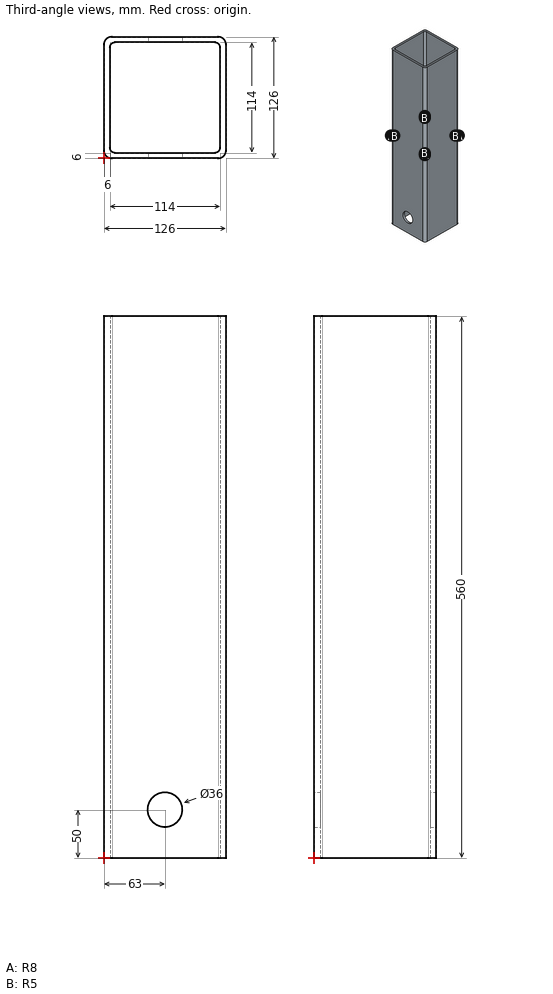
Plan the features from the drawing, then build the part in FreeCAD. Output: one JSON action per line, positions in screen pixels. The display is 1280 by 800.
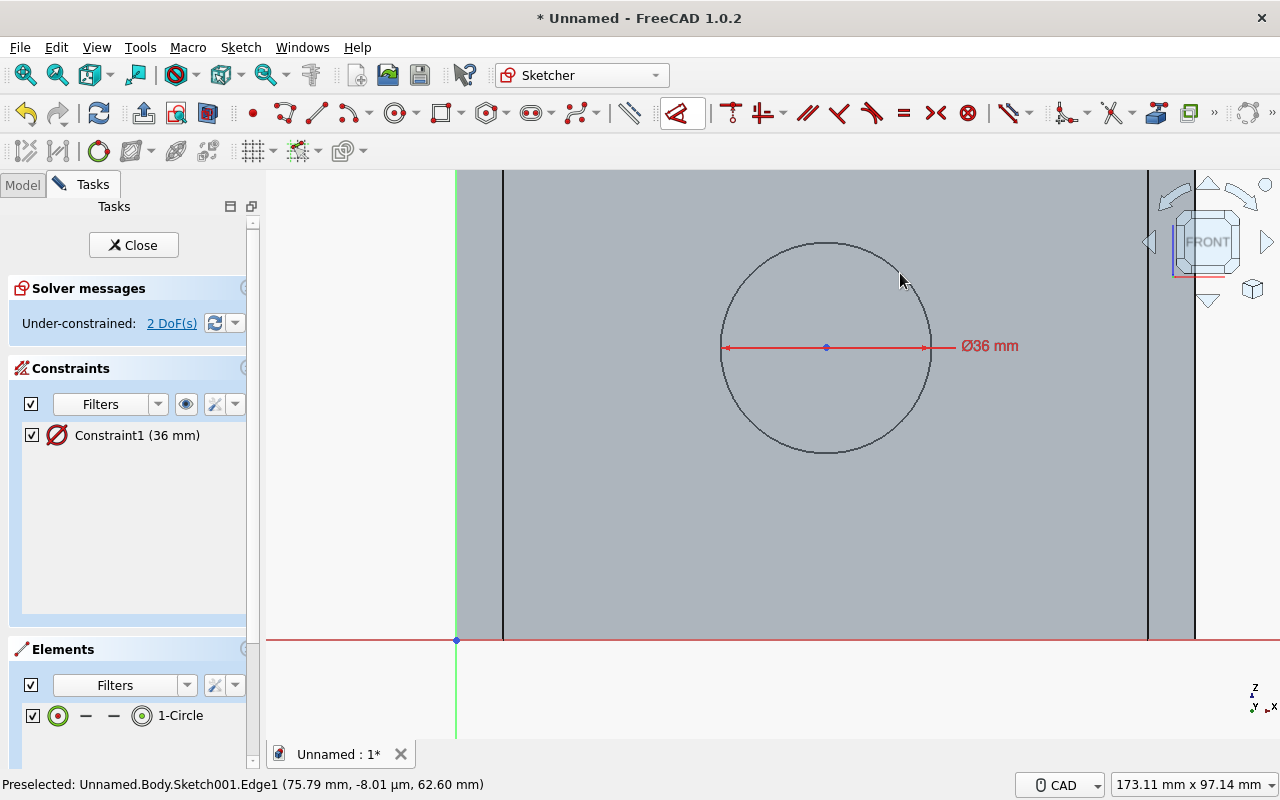
{"action": "left_click", "coordinate": [826, 348]}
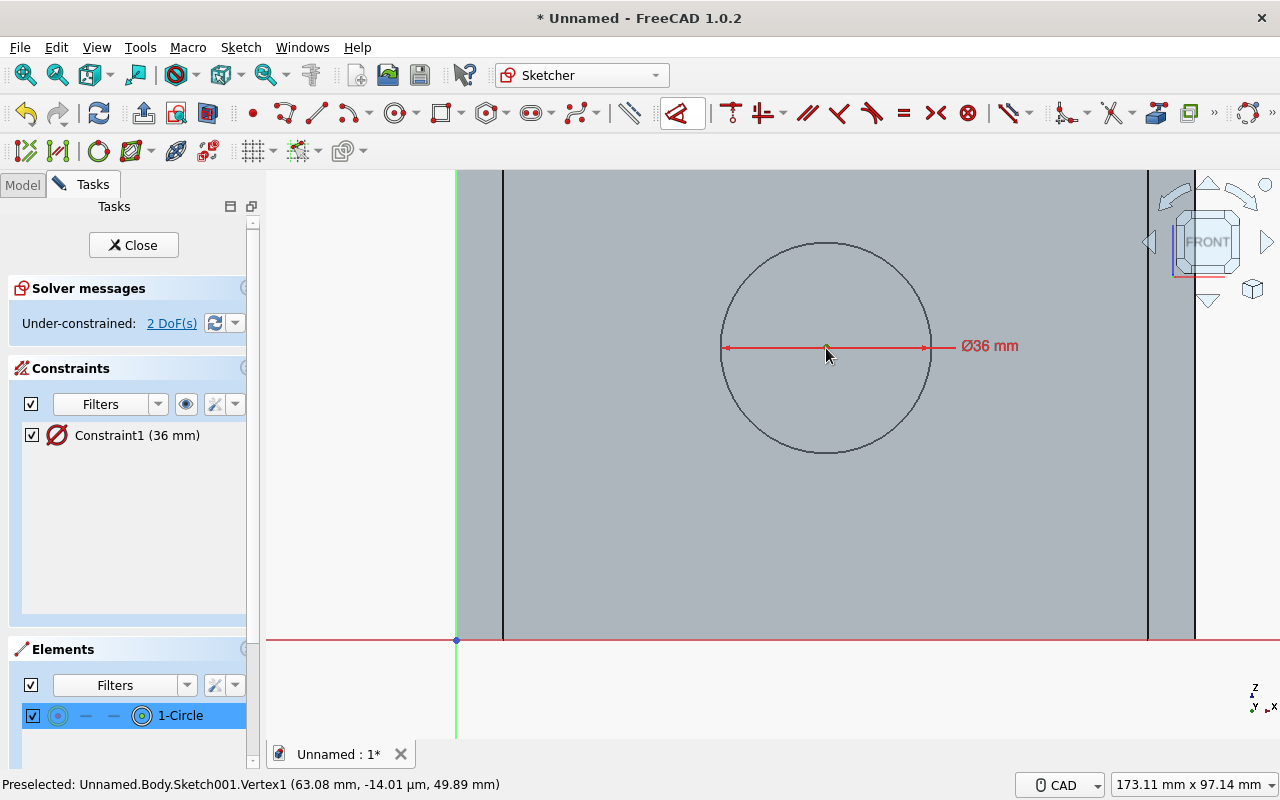
{"action": "left_click", "coordinate": [700, 114]}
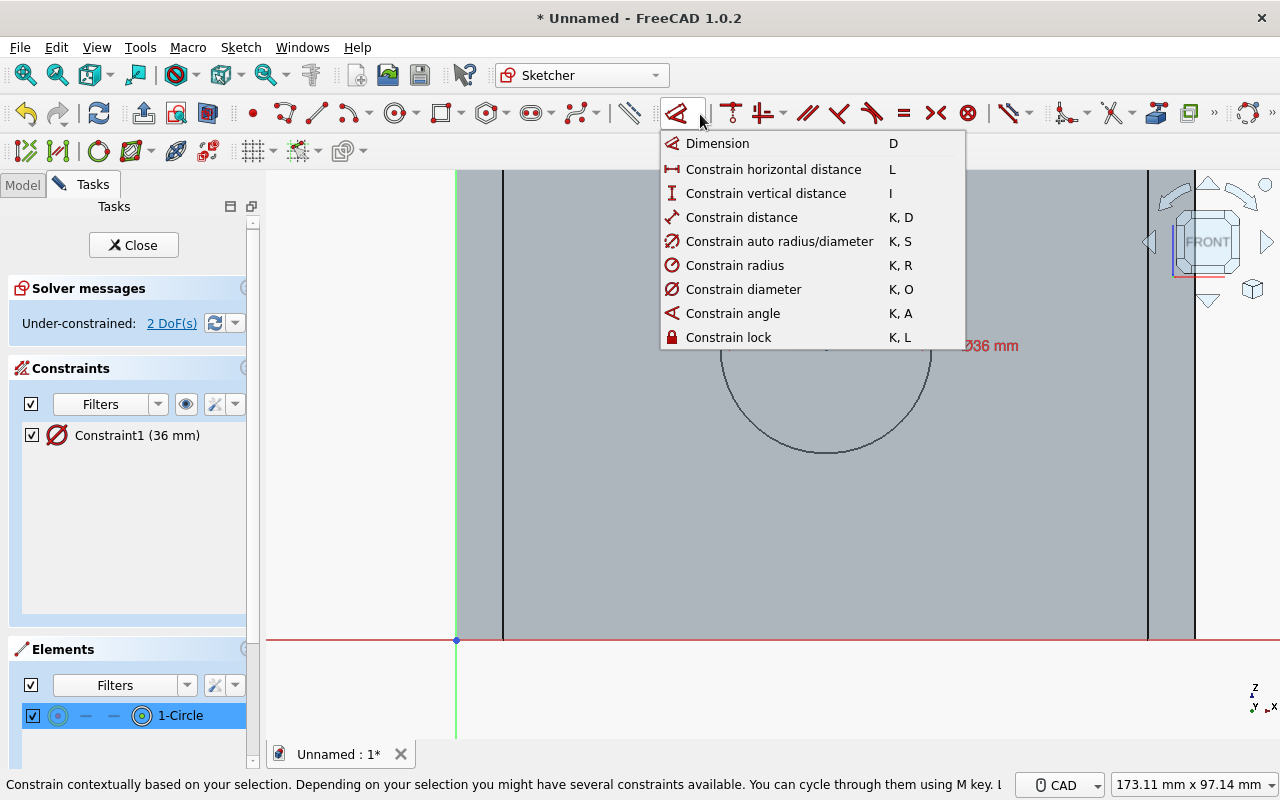
{"action": "left_click", "coordinate": [813, 169]}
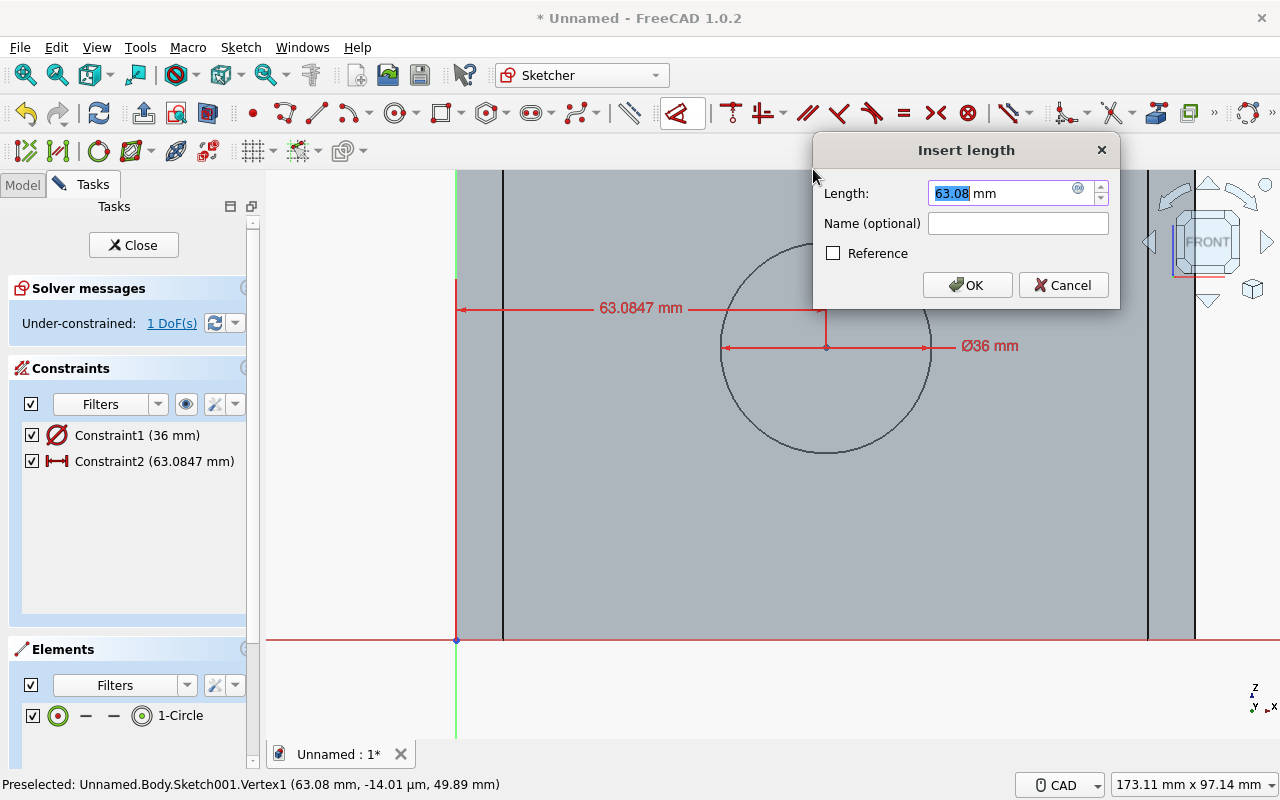
{"action": "type", "text": "63"}
{"action": "key", "text": "Return"}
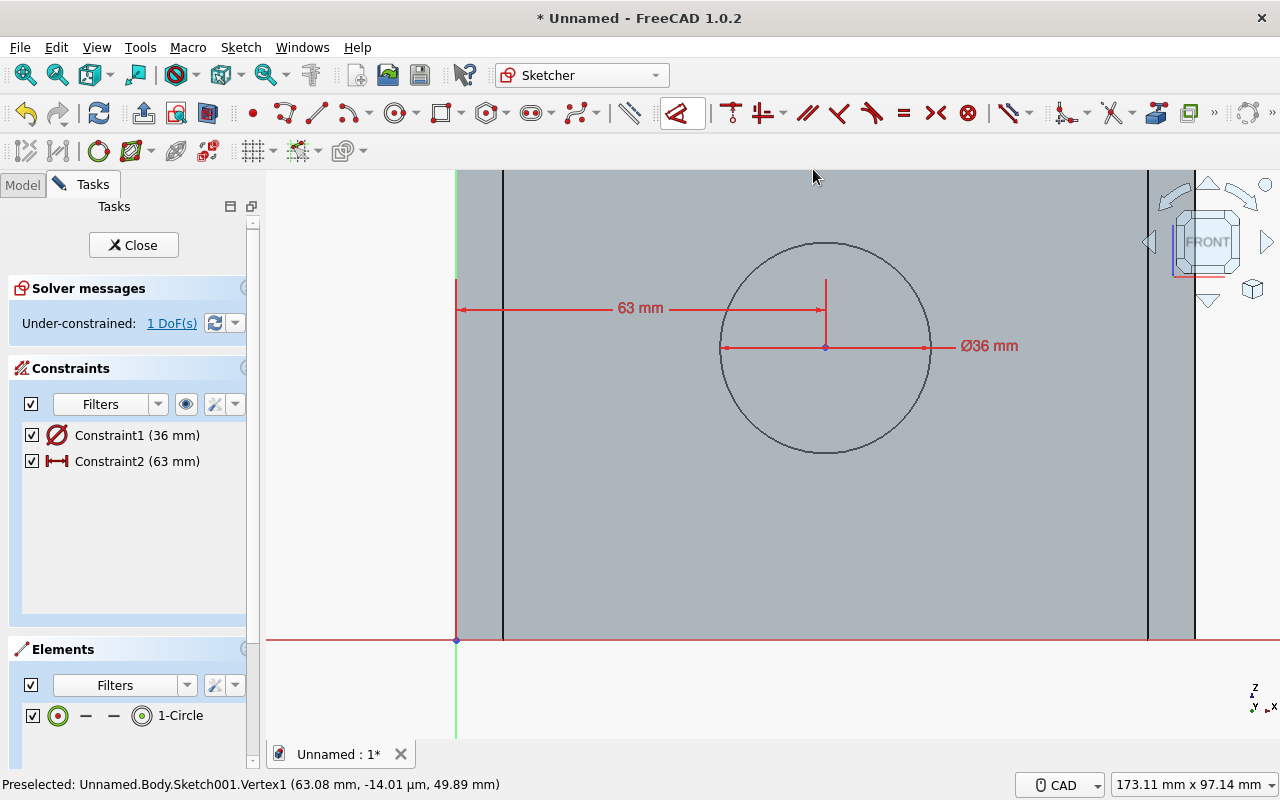
{"action": "left_click", "coordinate": [826, 348]}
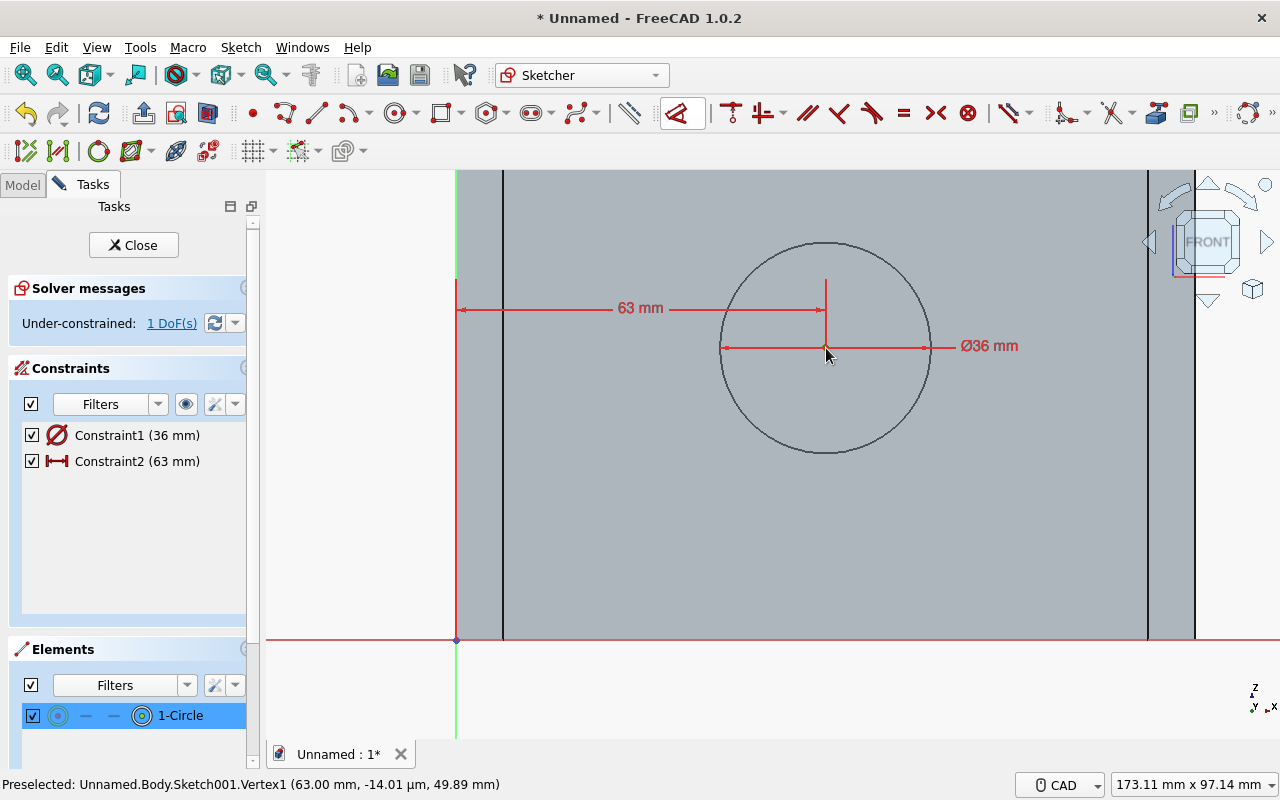
{"action": "key", "text": "i"}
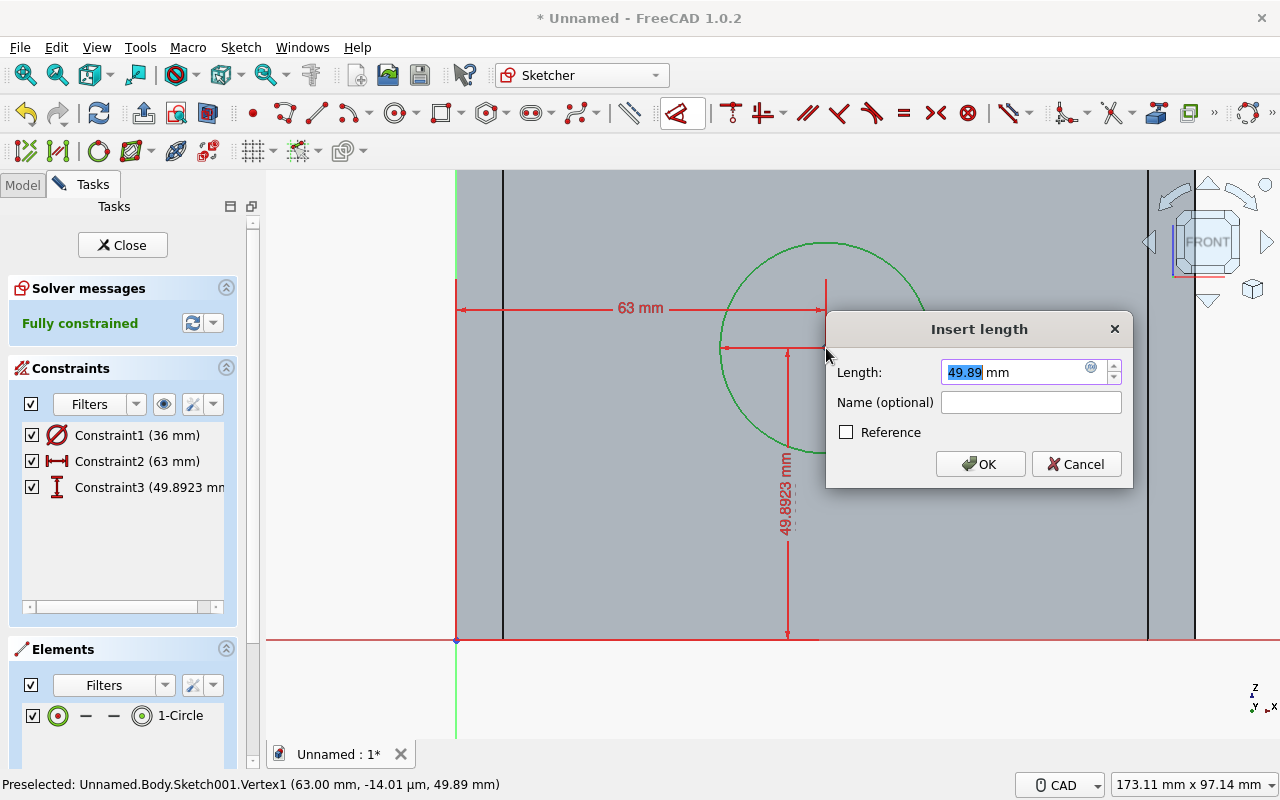
{"action": "type", "text": "50"}
{"action": "key", "text": "Return"}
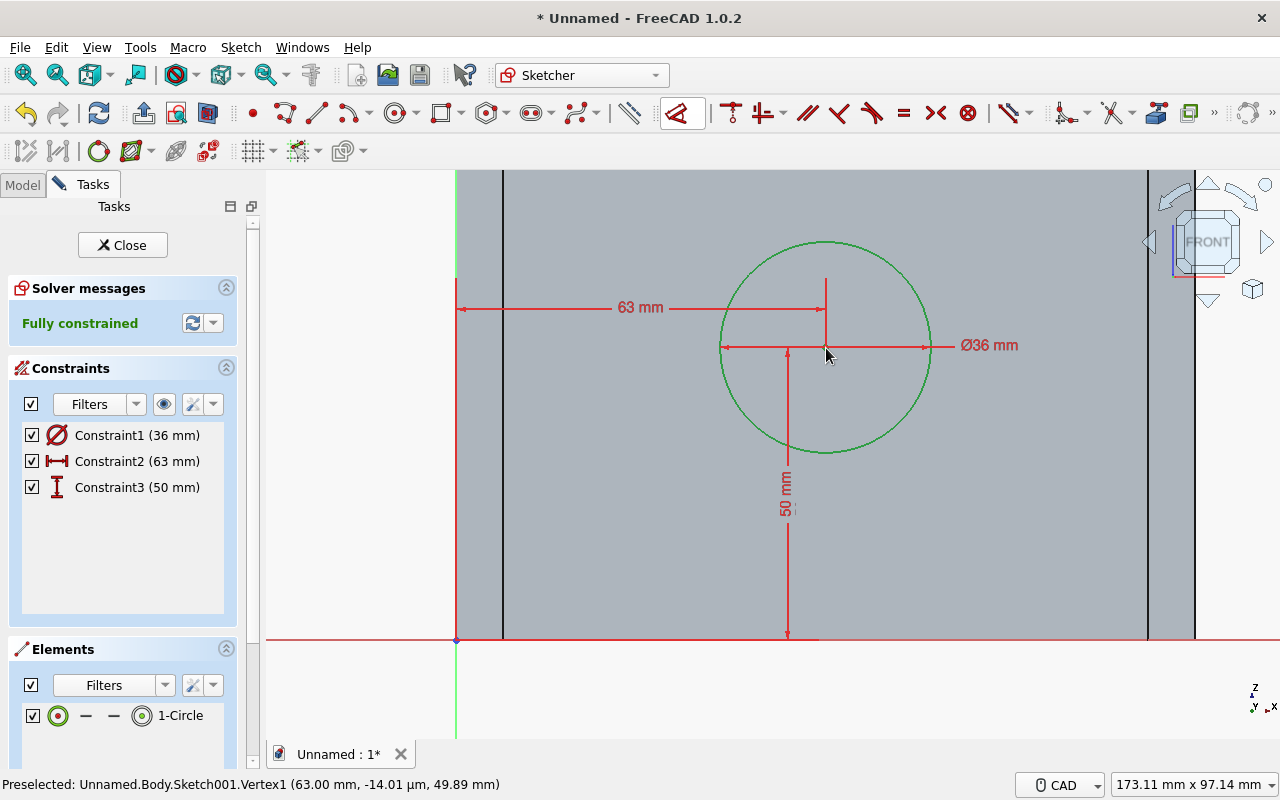
{"action": "left_click", "coordinate": [123, 245]}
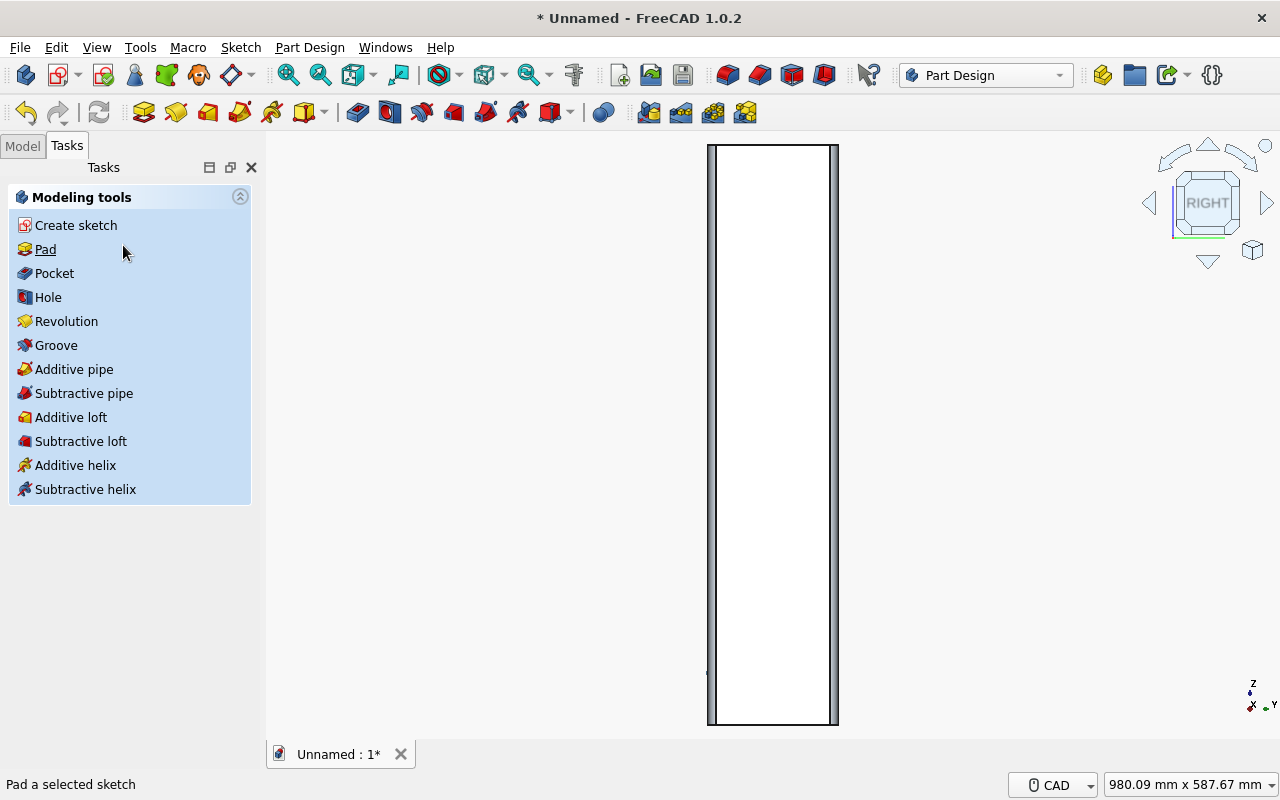
{"action": "left_click", "coordinate": [358, 112]}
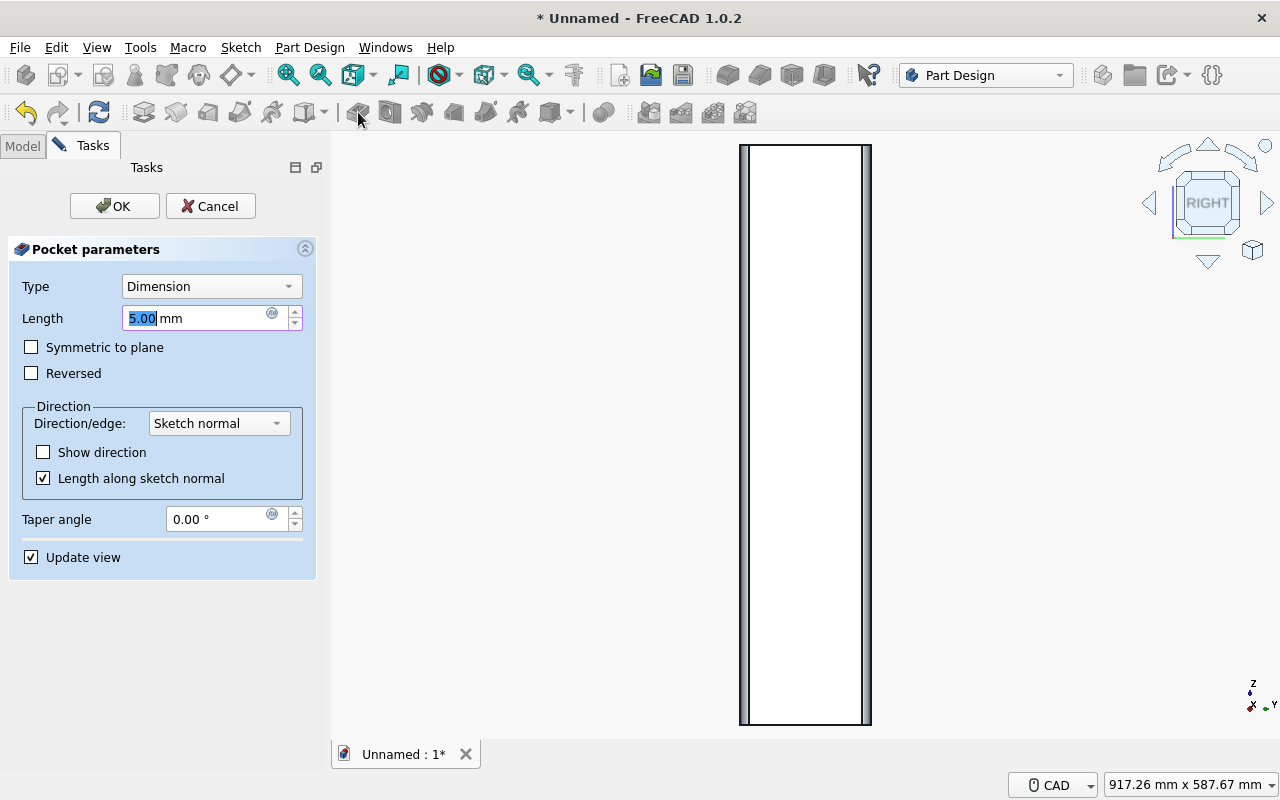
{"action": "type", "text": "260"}
{"action": "key", "text": "Tab"}